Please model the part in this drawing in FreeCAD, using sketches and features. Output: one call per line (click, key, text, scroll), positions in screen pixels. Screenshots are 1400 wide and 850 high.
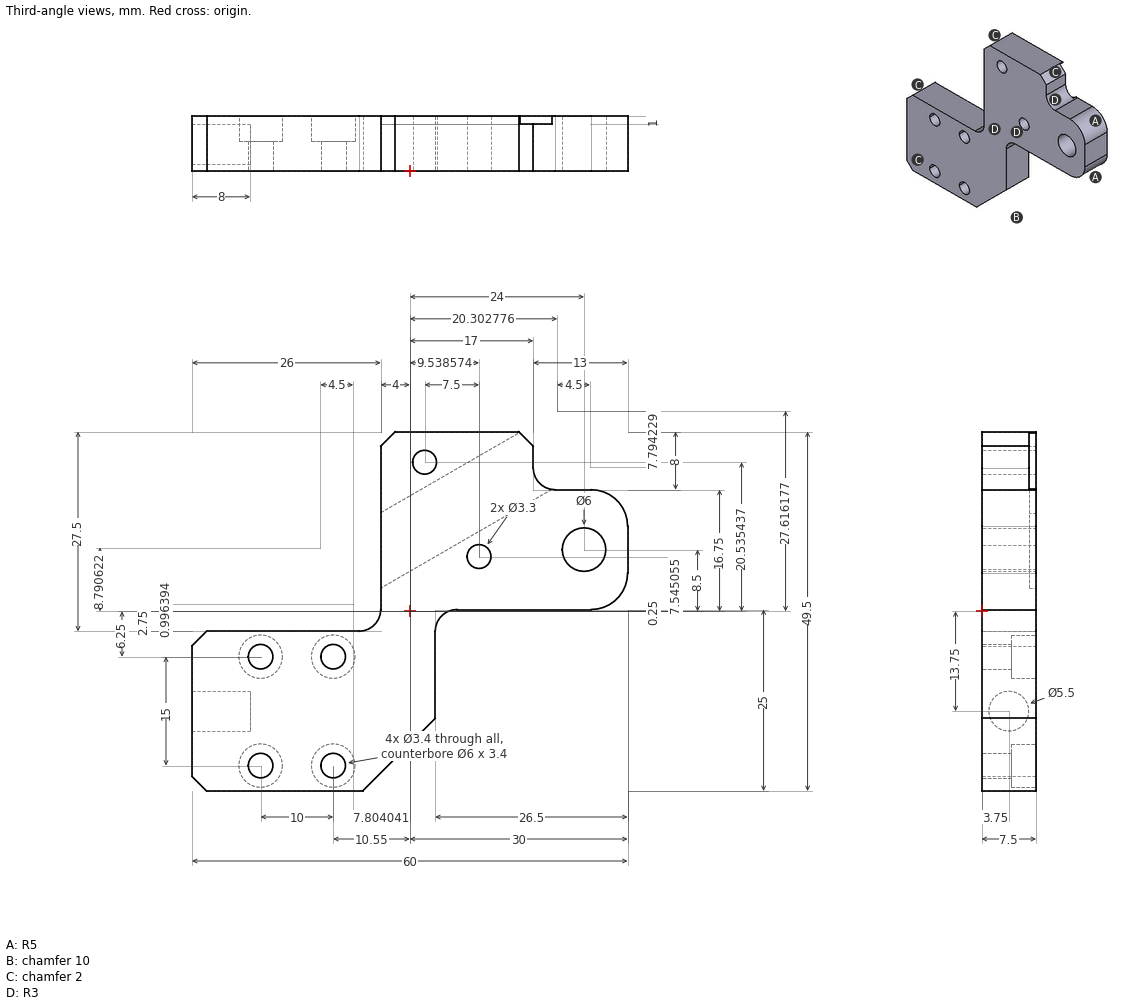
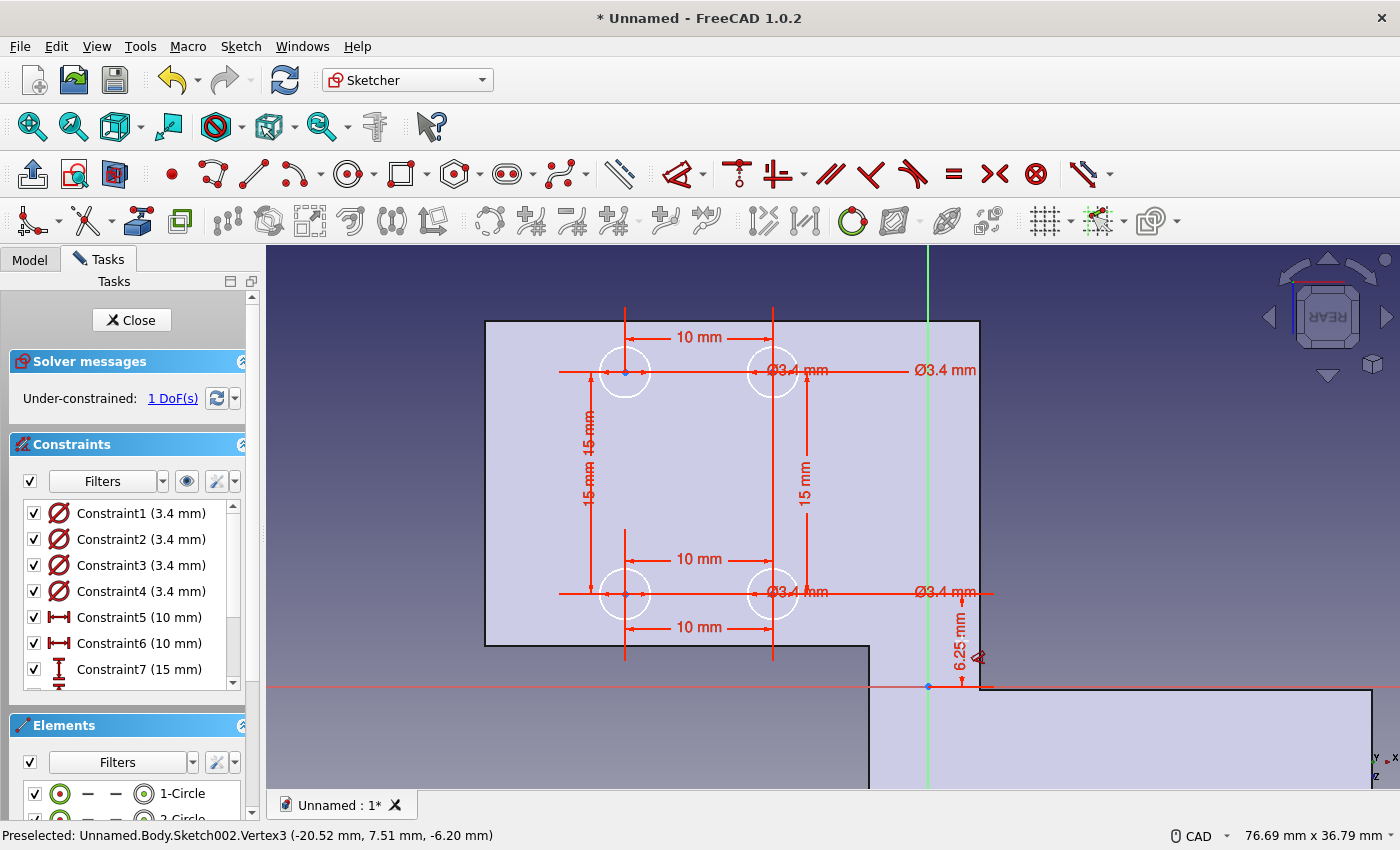
click(773, 372)
click(851, 721)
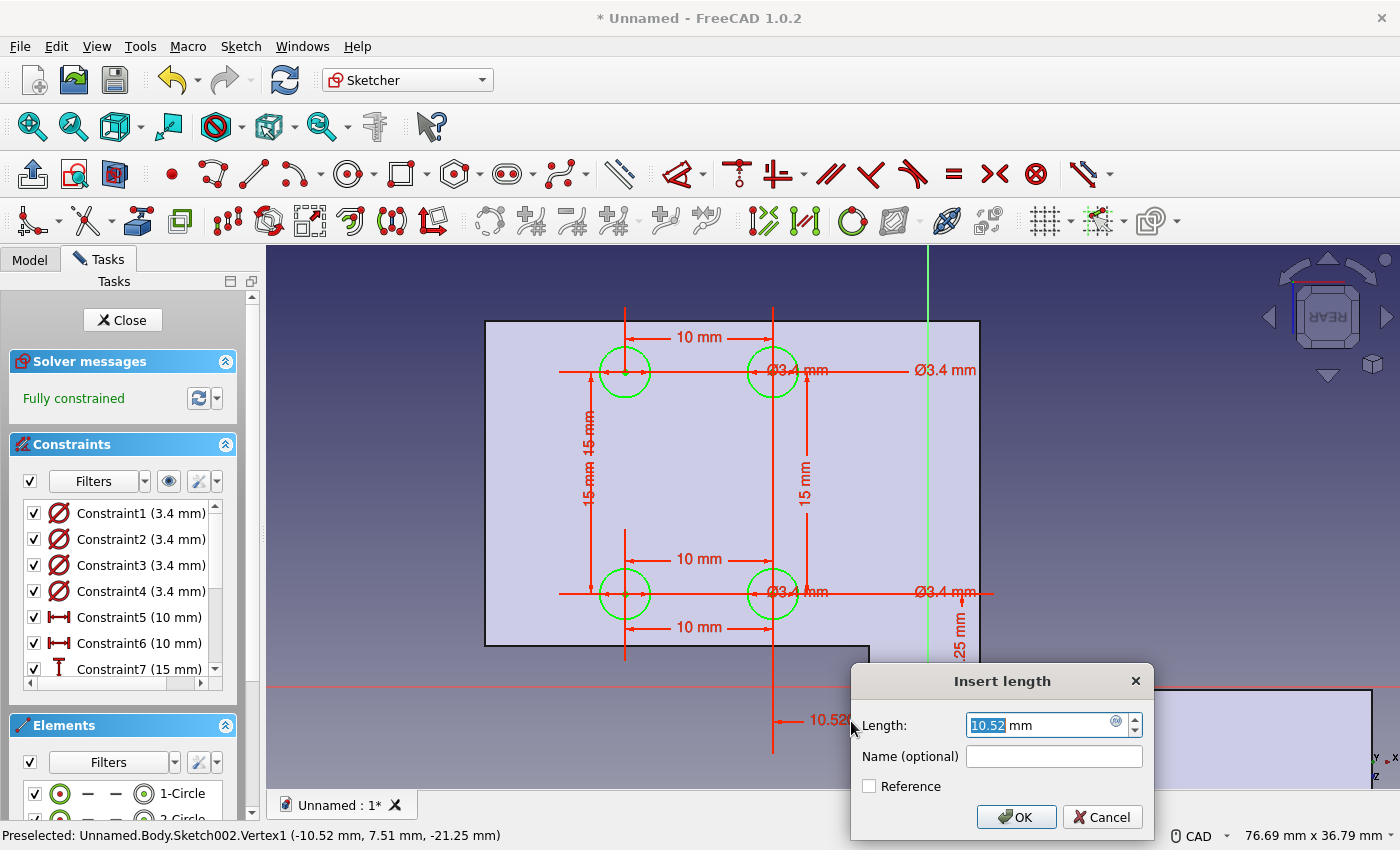
text(10.55)
key(Return)
key(Escape)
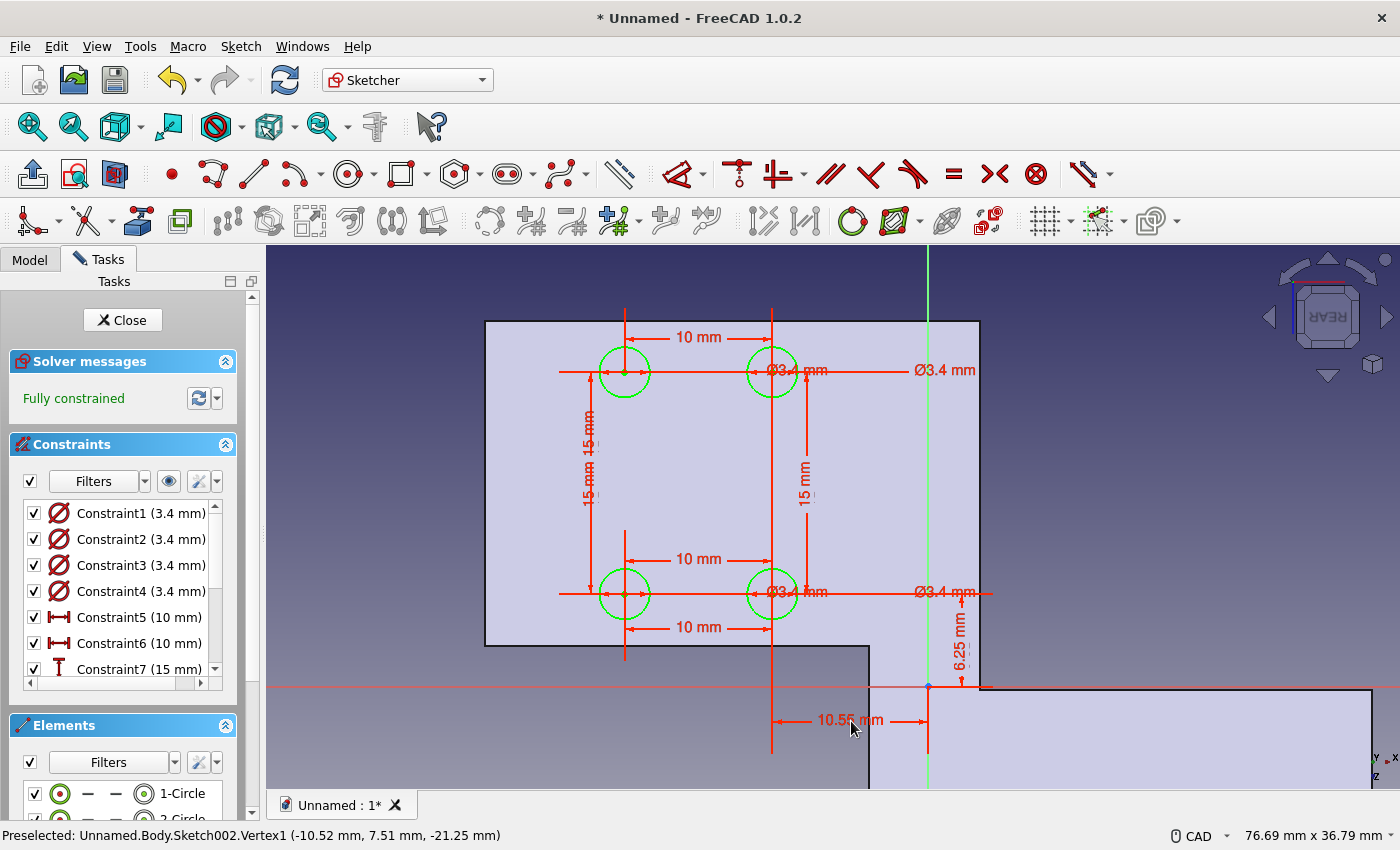
click(123, 320)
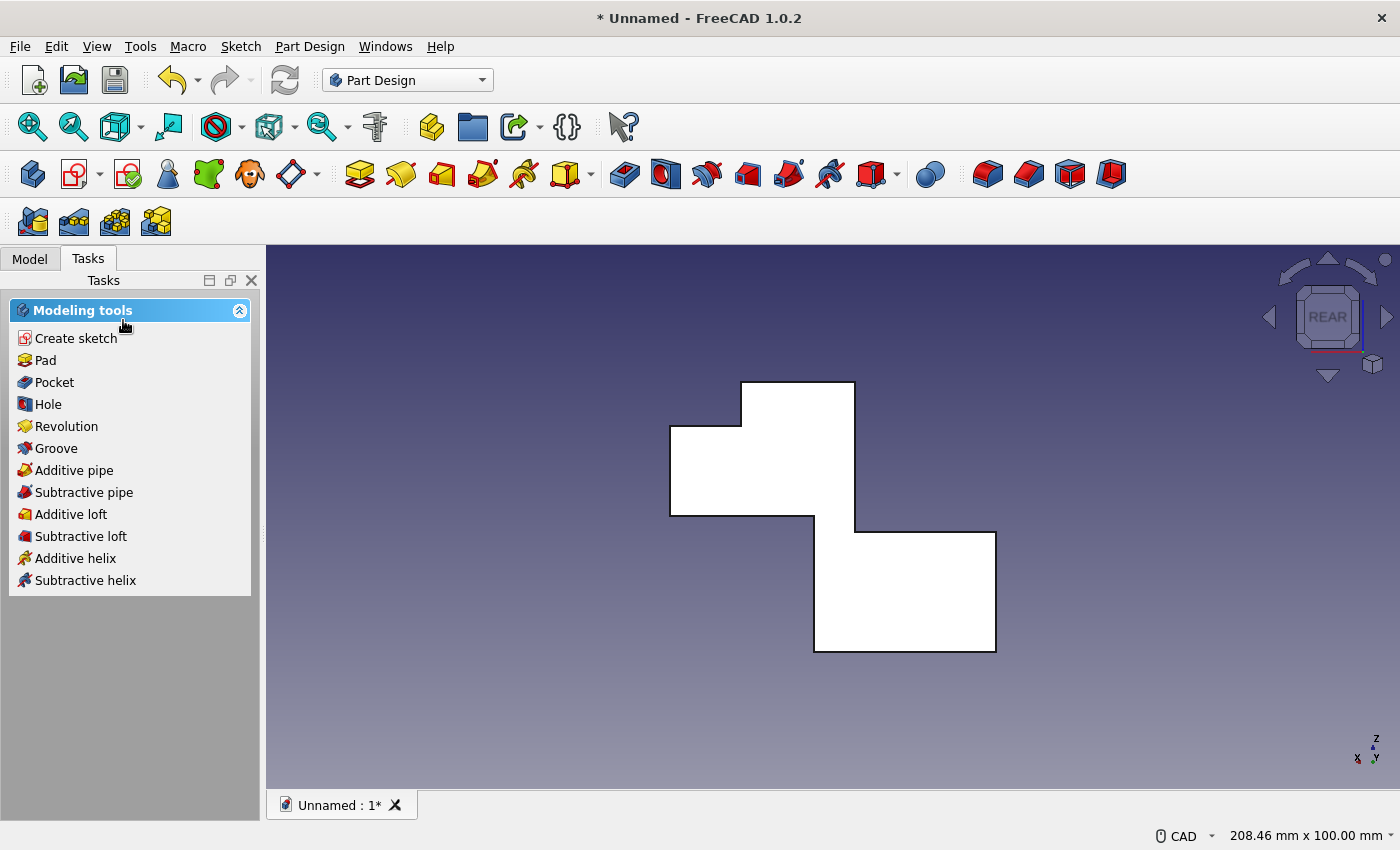
click(666, 174)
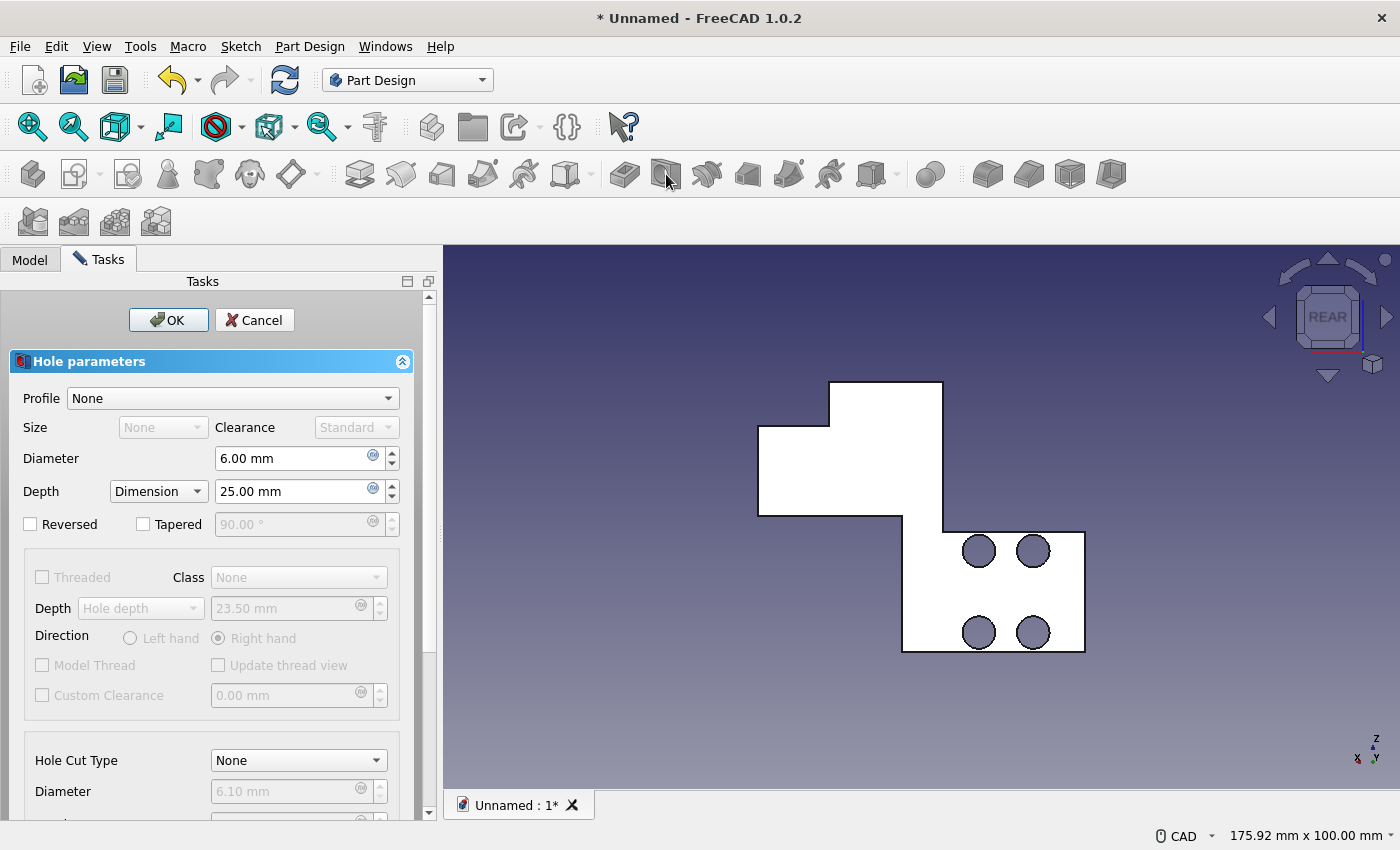
triple_click(300, 458)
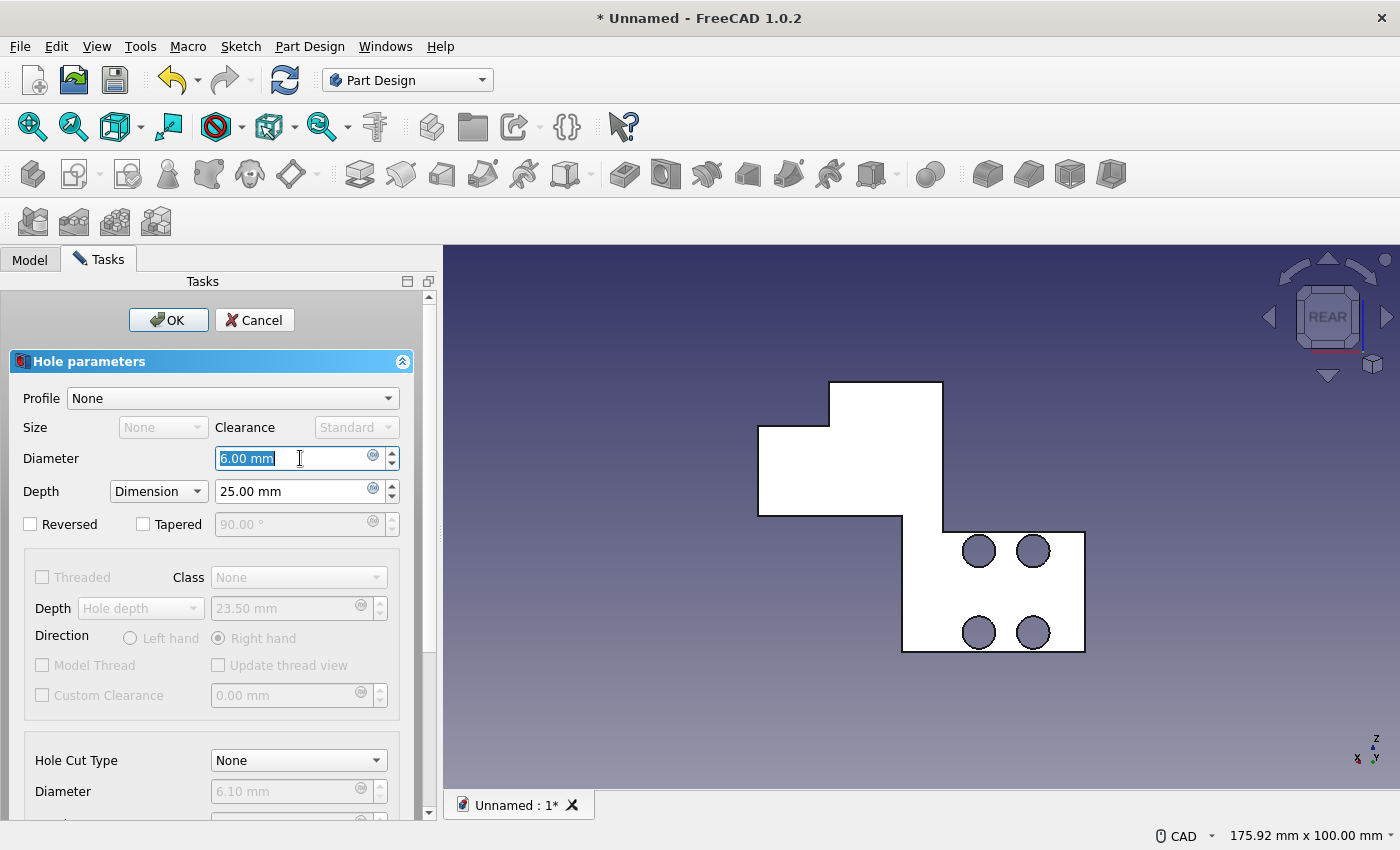
text(3.4)
key(Tab)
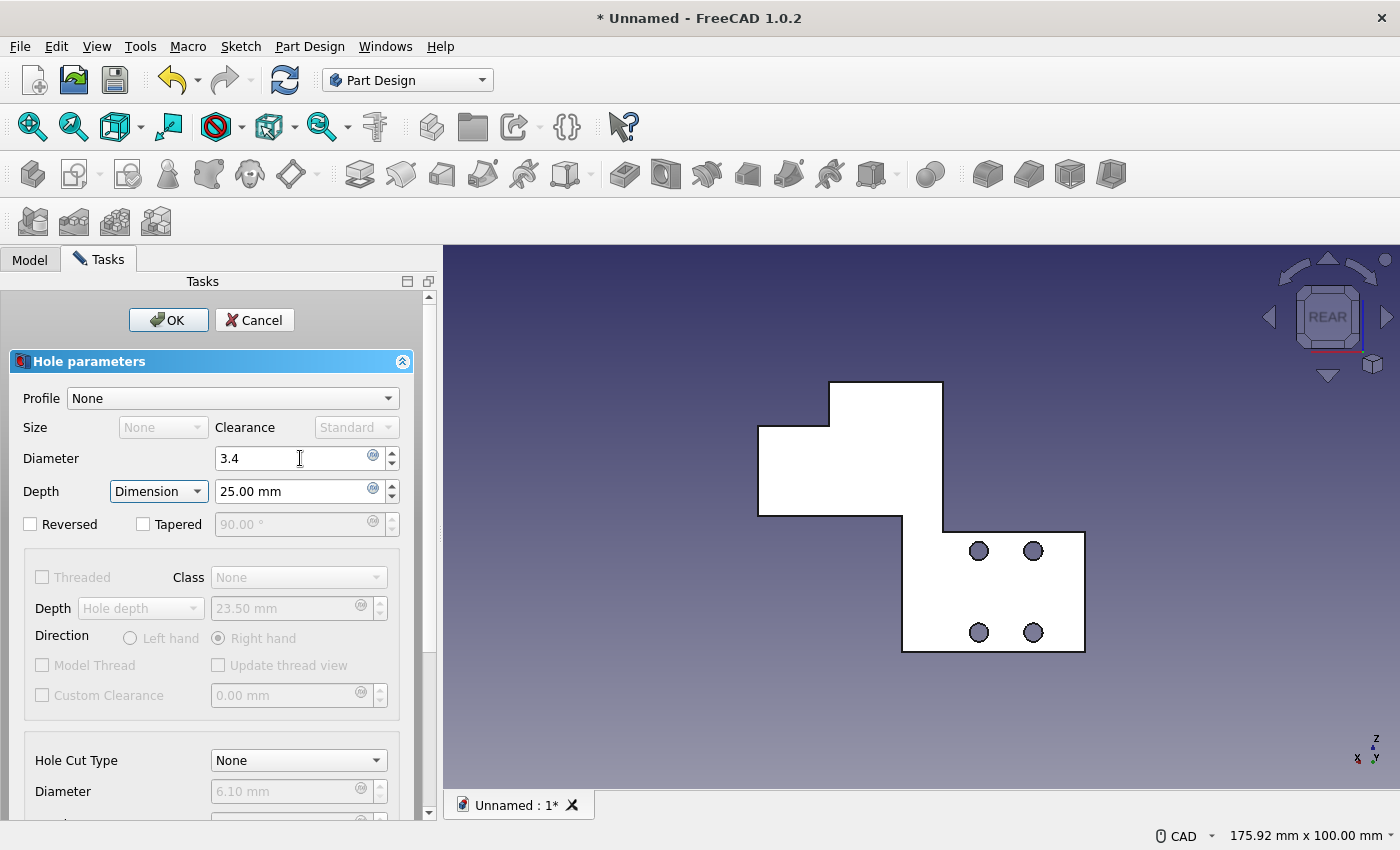
click(160, 492)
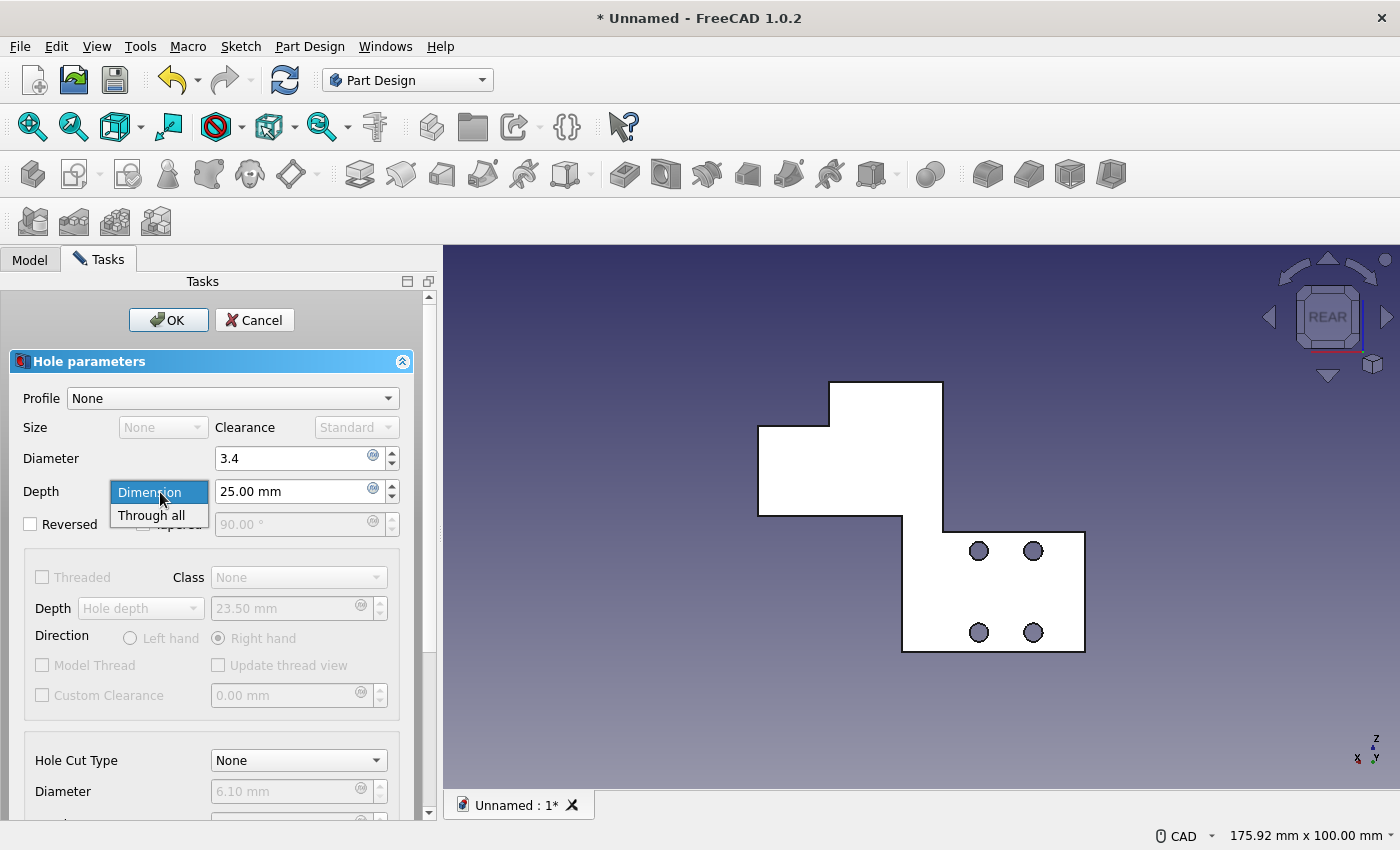
click(158, 516)